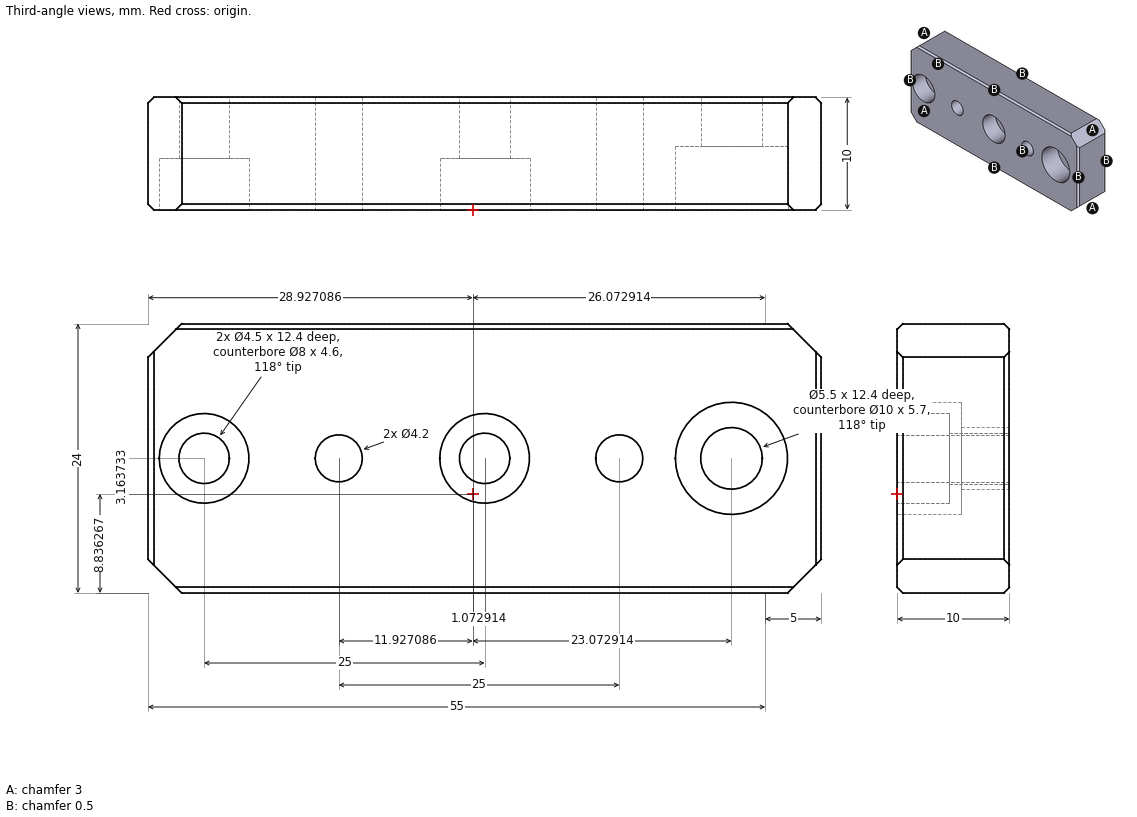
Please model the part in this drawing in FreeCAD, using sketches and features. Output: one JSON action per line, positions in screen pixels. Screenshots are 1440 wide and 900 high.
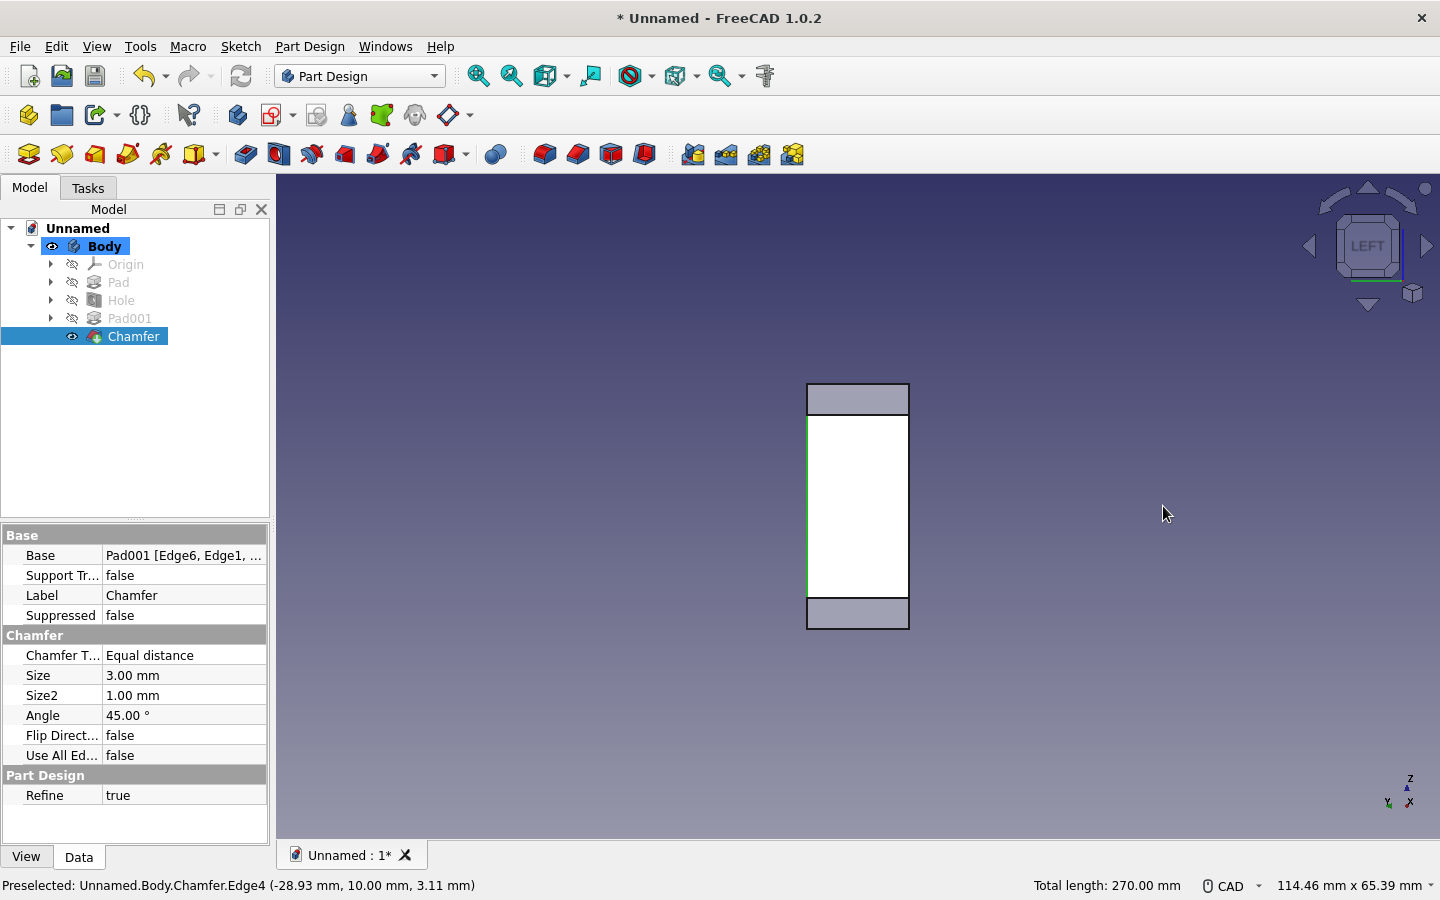
{"action": "left_click", "coordinate": [909, 505], "text": "ctrl"}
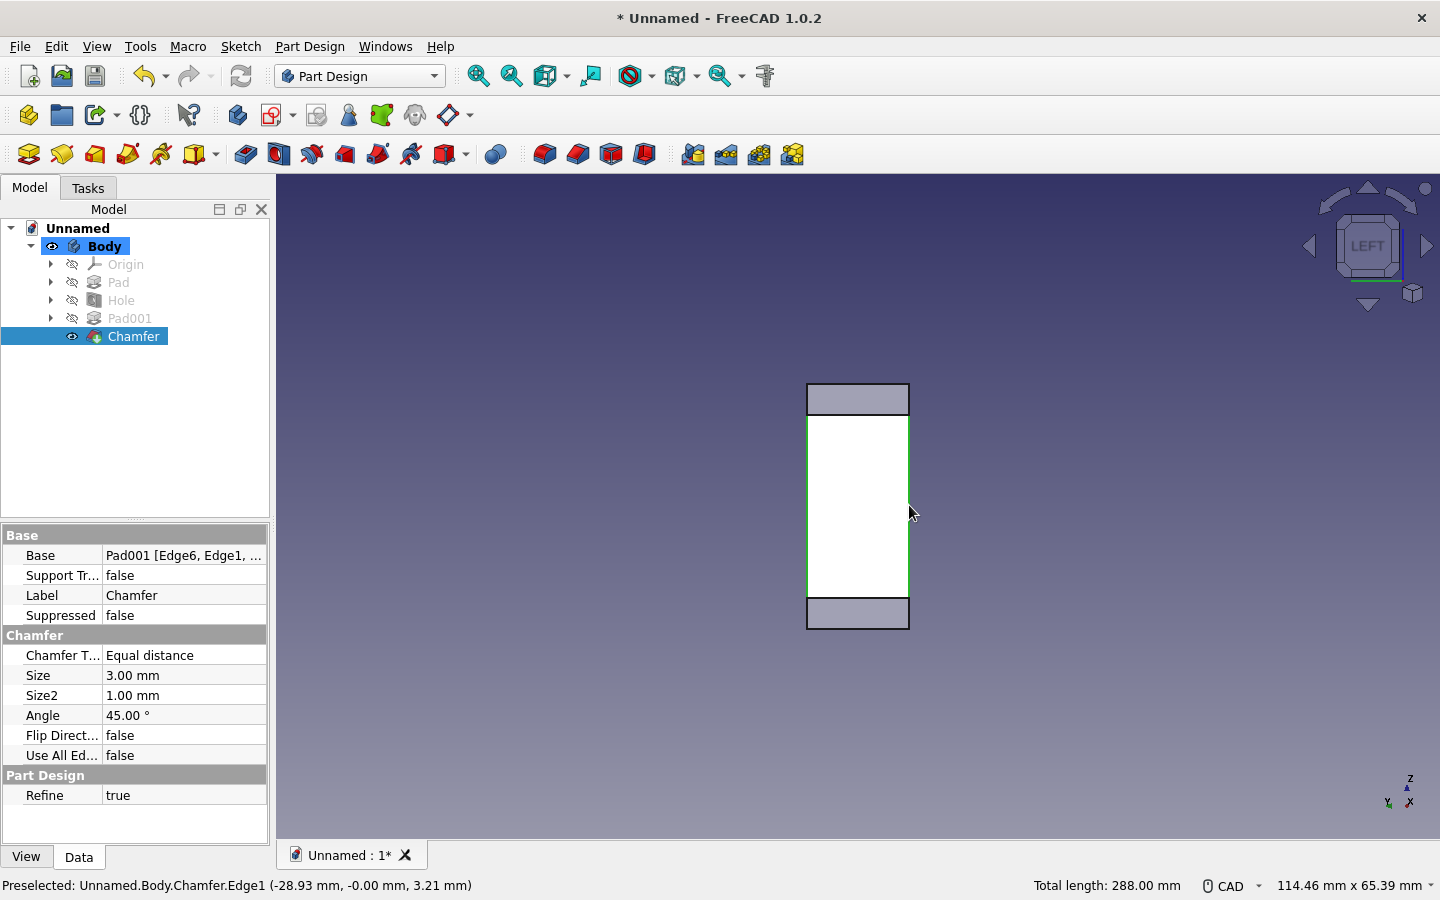
{"action": "left_click", "coordinate": [578, 154]}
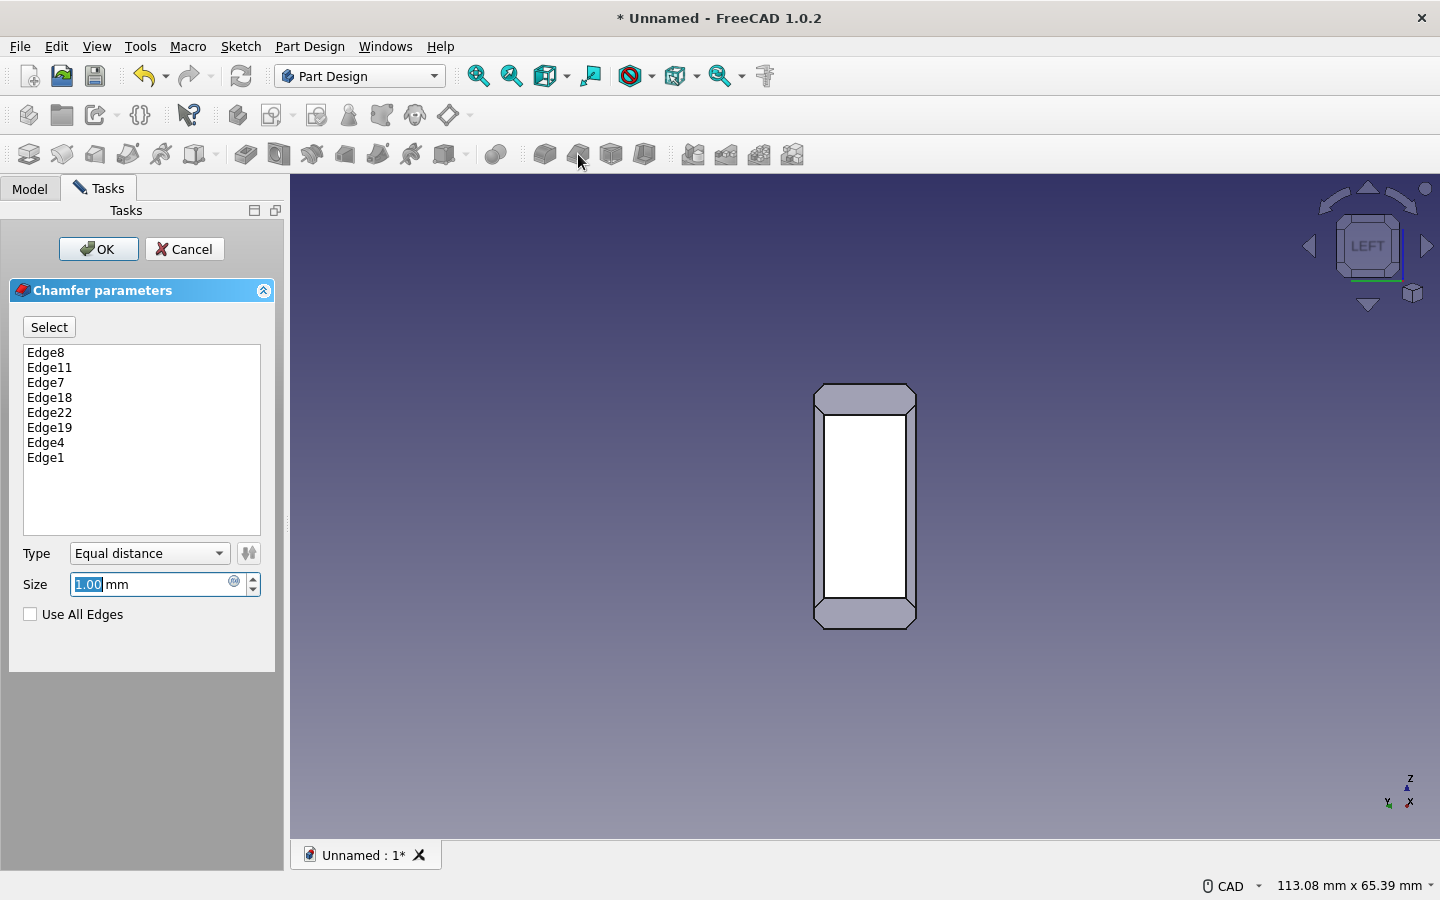
{"action": "type", "text": "0.5"}
{"action": "key", "text": "Tab"}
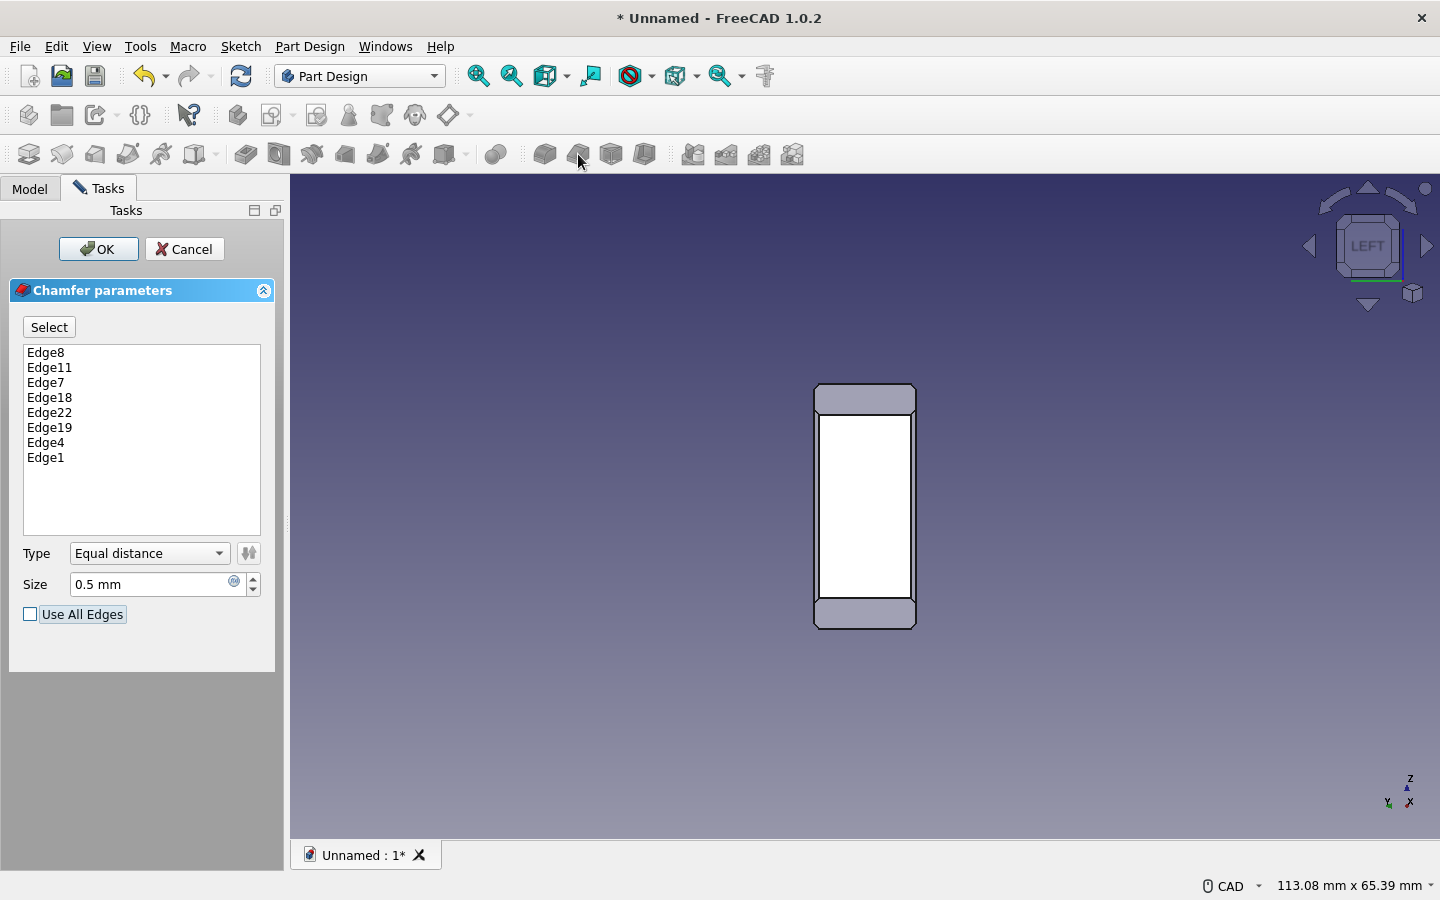
{"action": "left_click", "coordinate": [99, 249]}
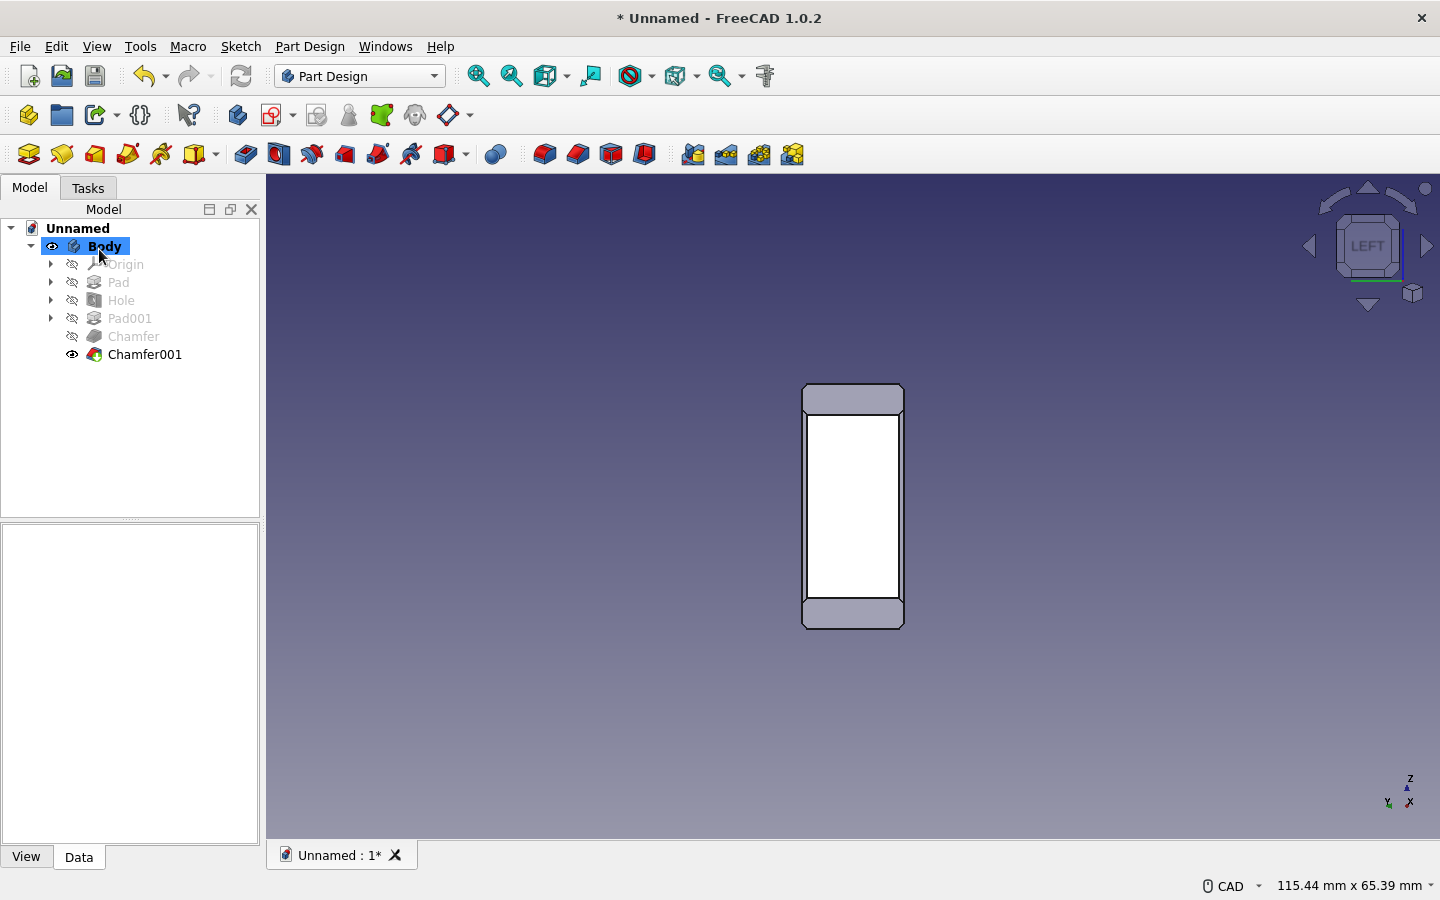
{"action": "left_click", "coordinate": [479, 76]}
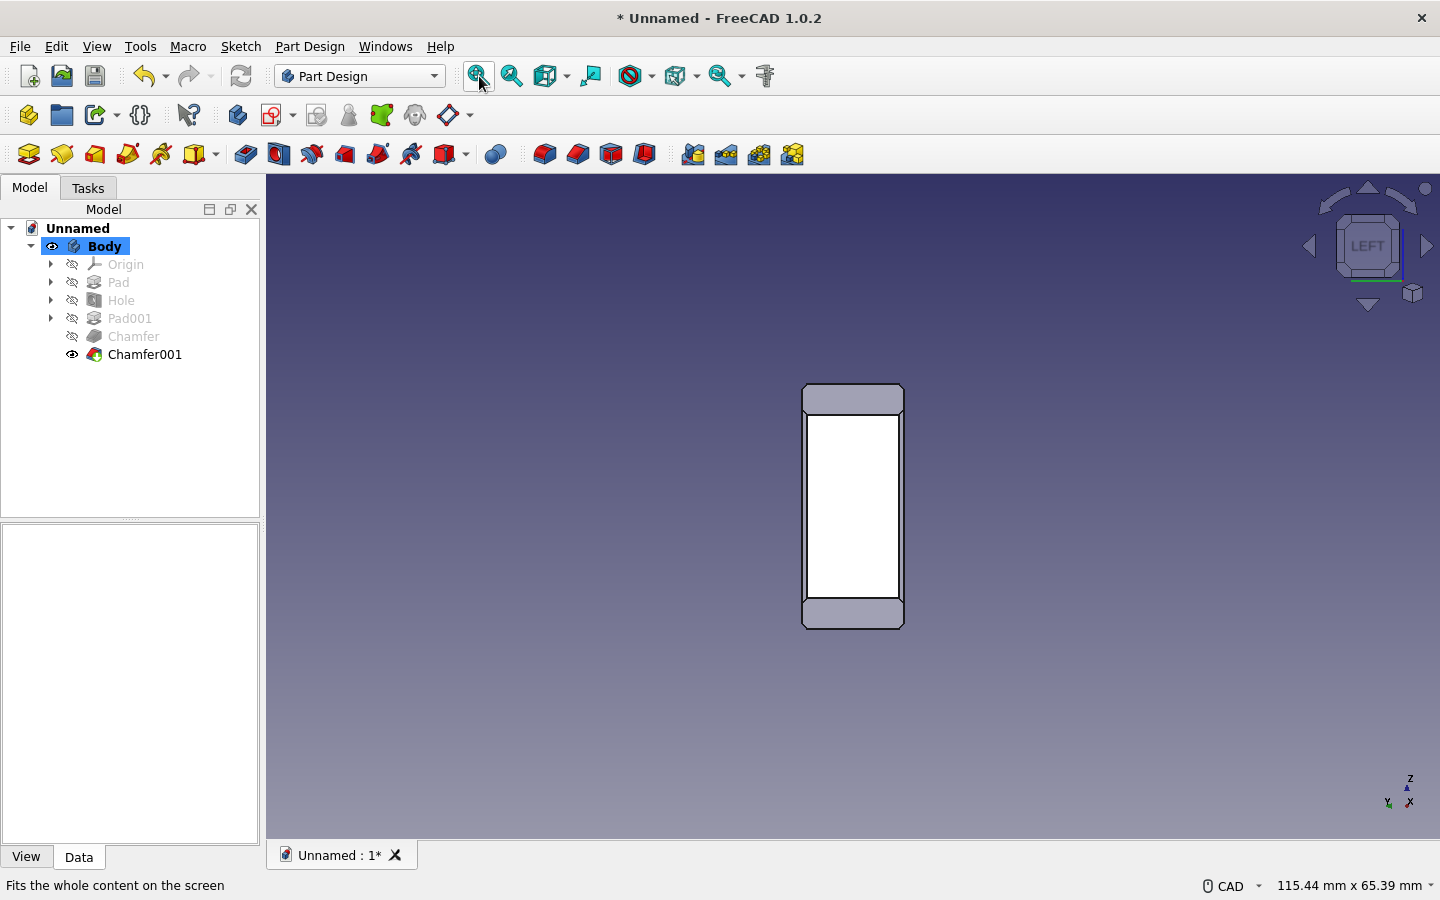
{"action": "key", "text": "0"}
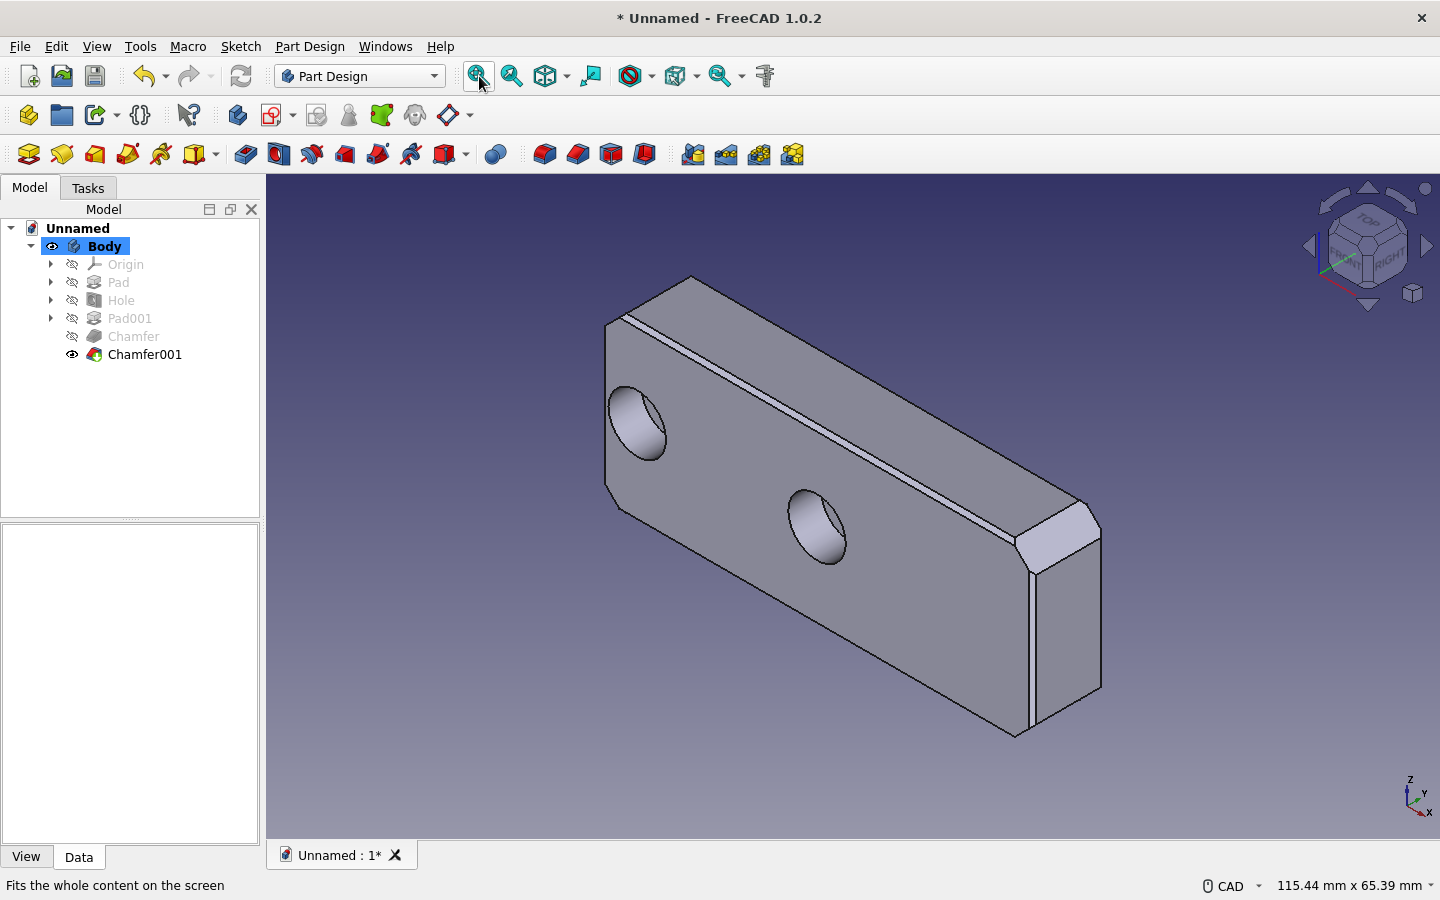
{"action": "left_click", "coordinate": [938, 596]}